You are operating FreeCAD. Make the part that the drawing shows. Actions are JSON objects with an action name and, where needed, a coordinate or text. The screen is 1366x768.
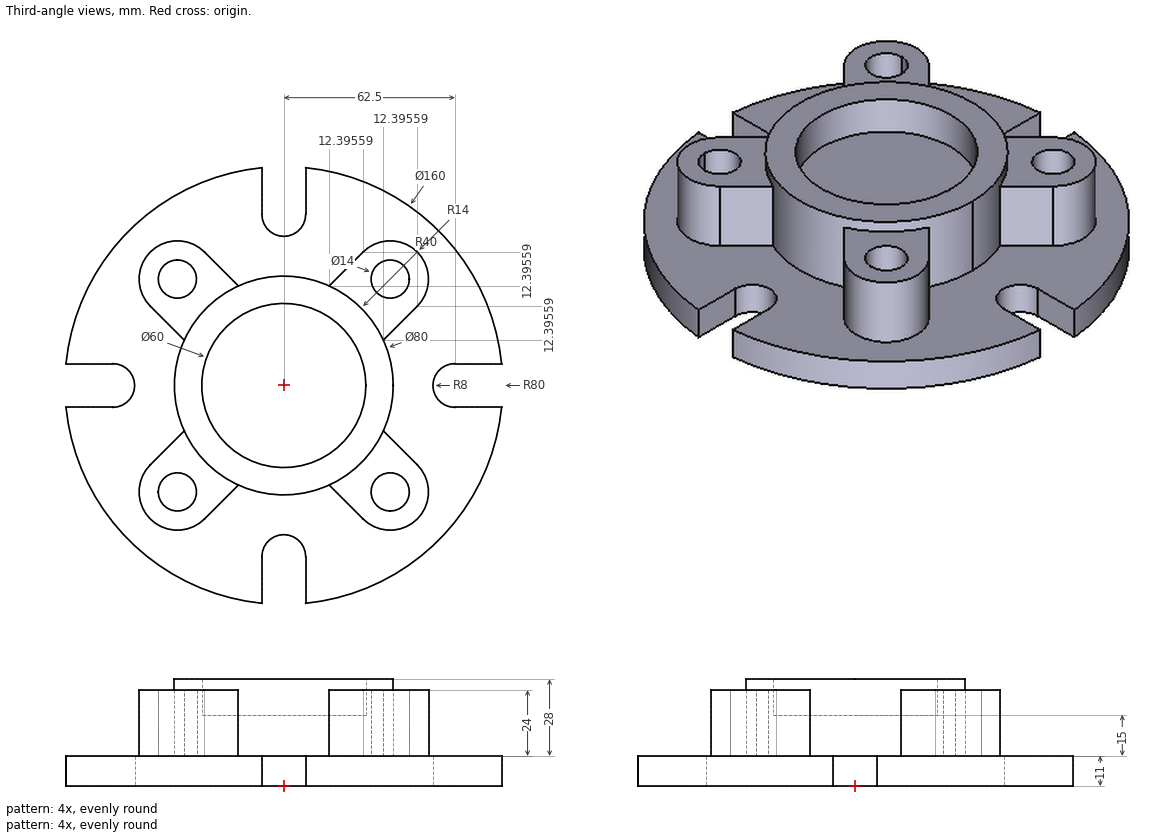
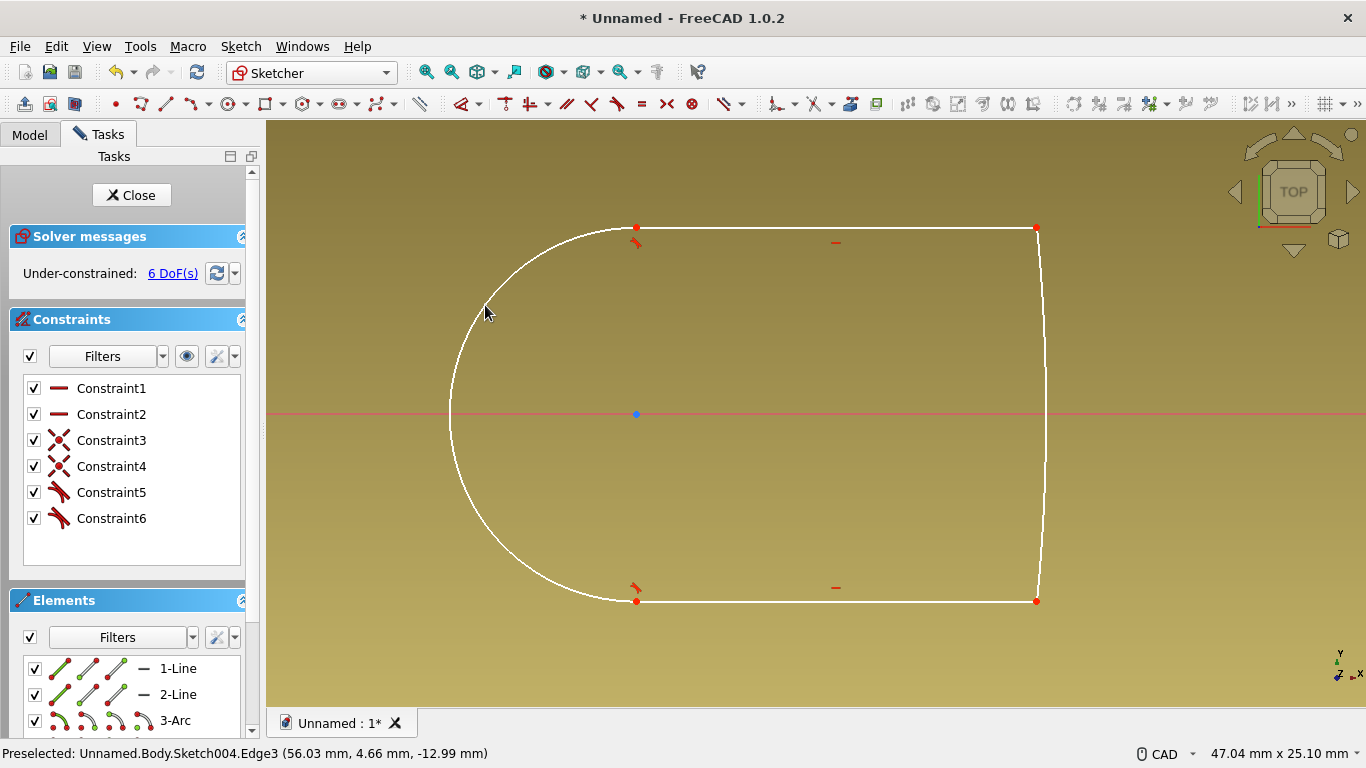
{"action": "scroll", "coordinate": [1125, 413], "scroll_direction": "down", "scroll_amount": 5}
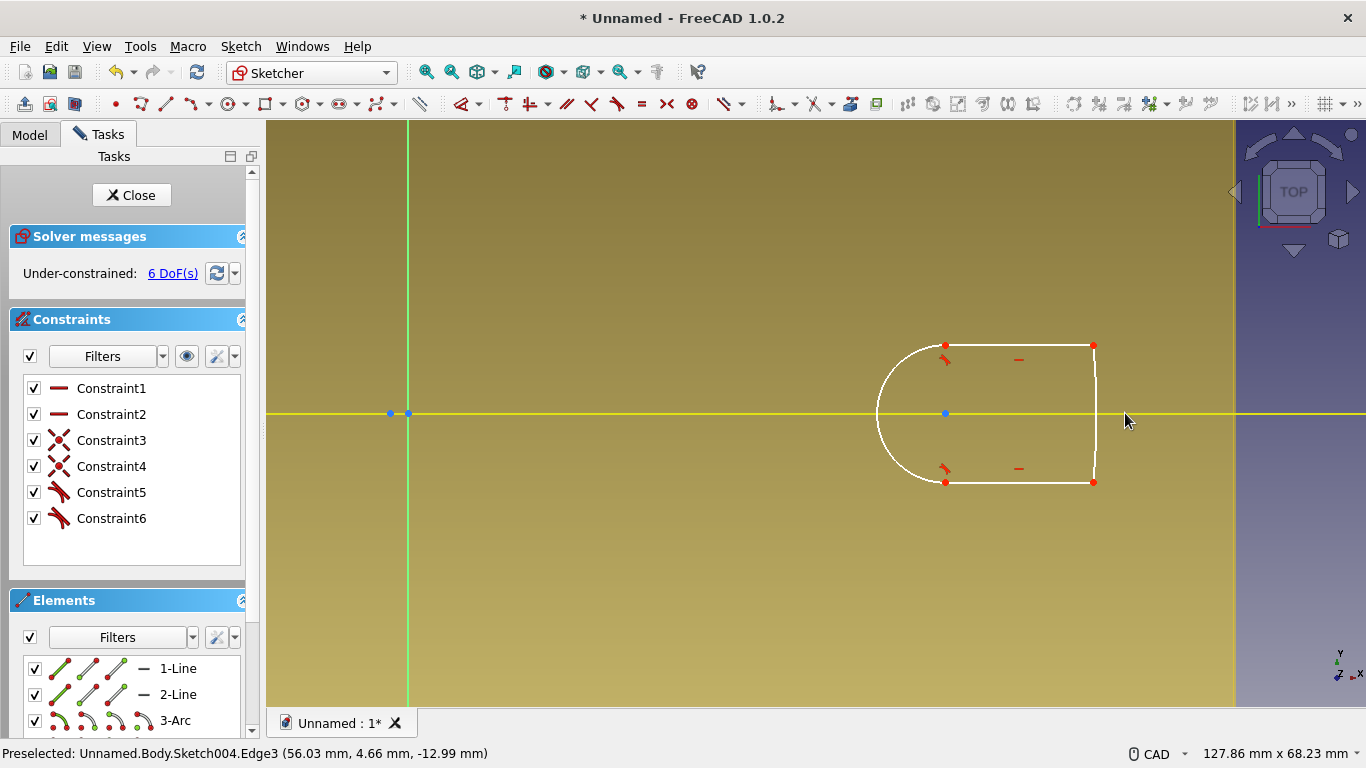
{"action": "left_click_drag", "start_coordinate": [380, 404], "coordinate": [418, 424]}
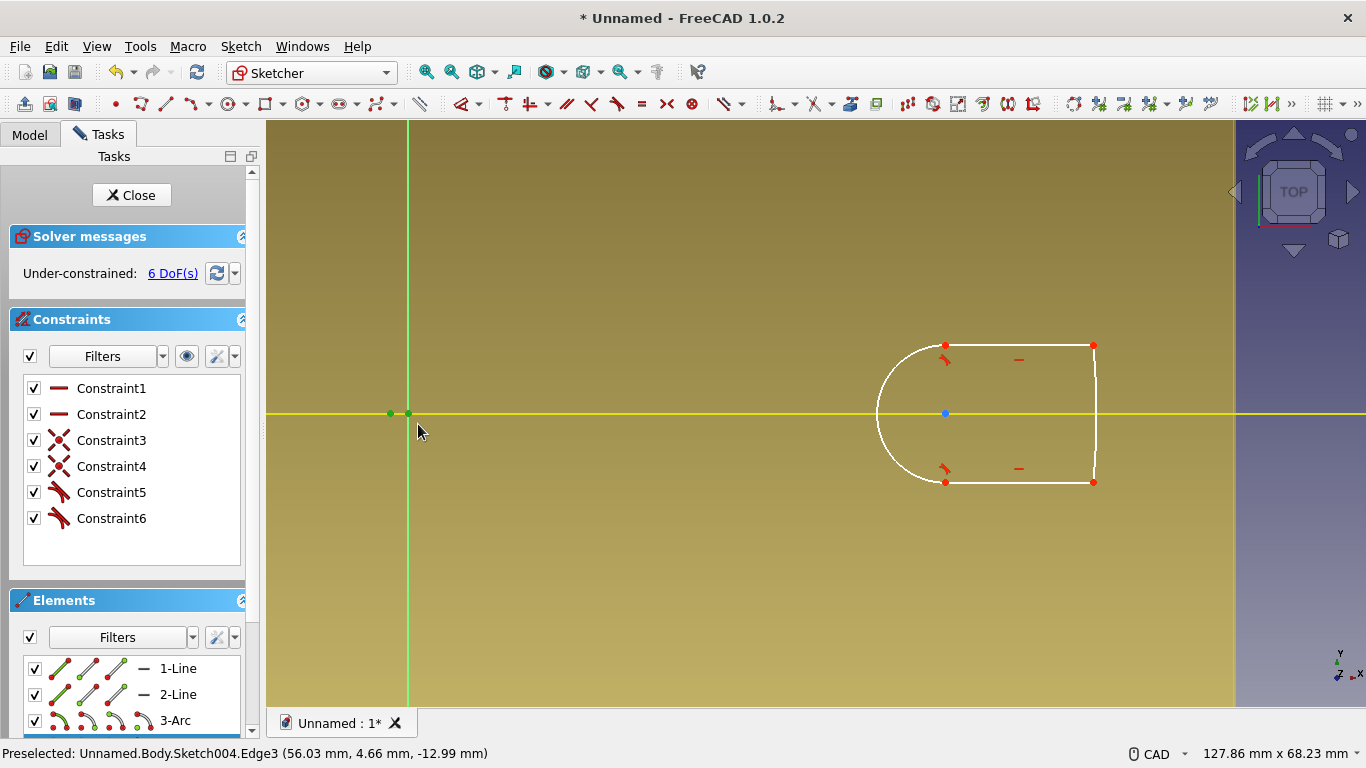
{"action": "key", "text": "c"}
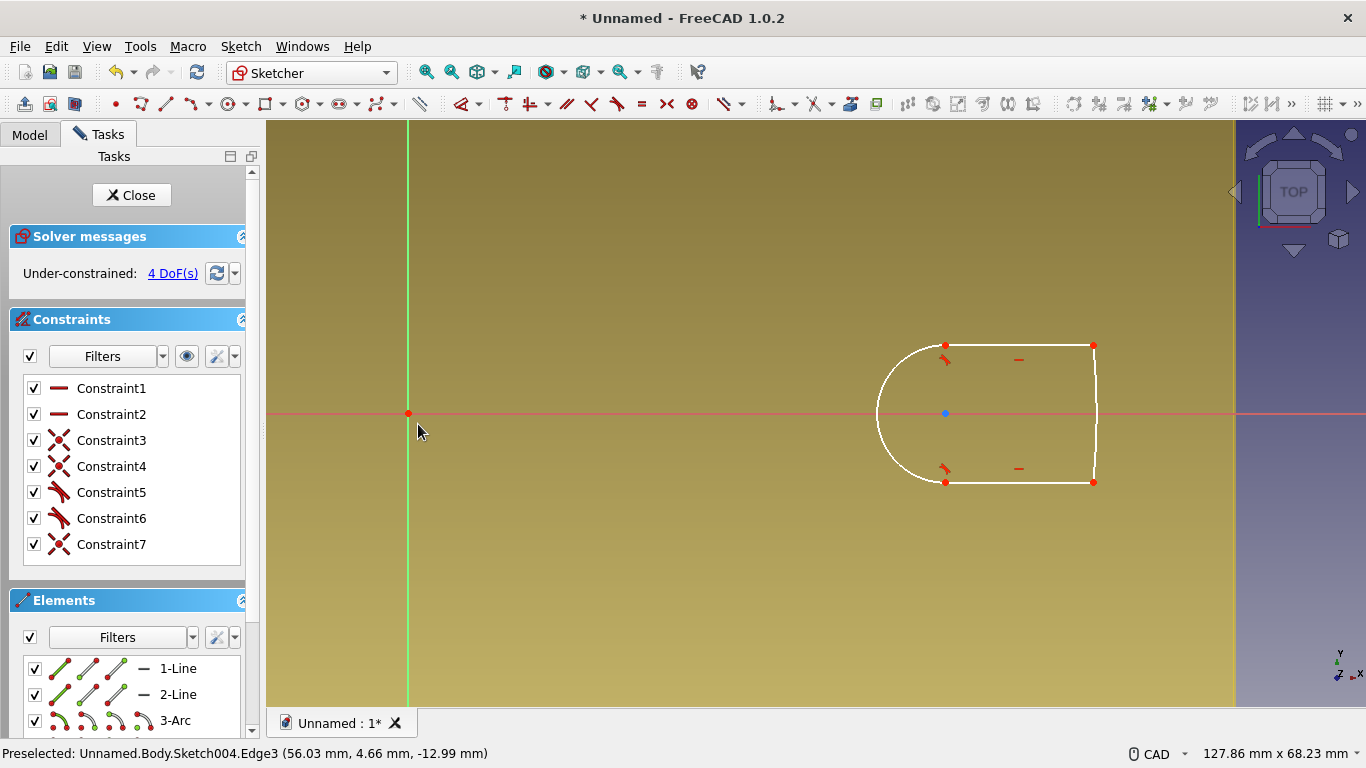
{"action": "left_click", "coordinate": [946, 414]}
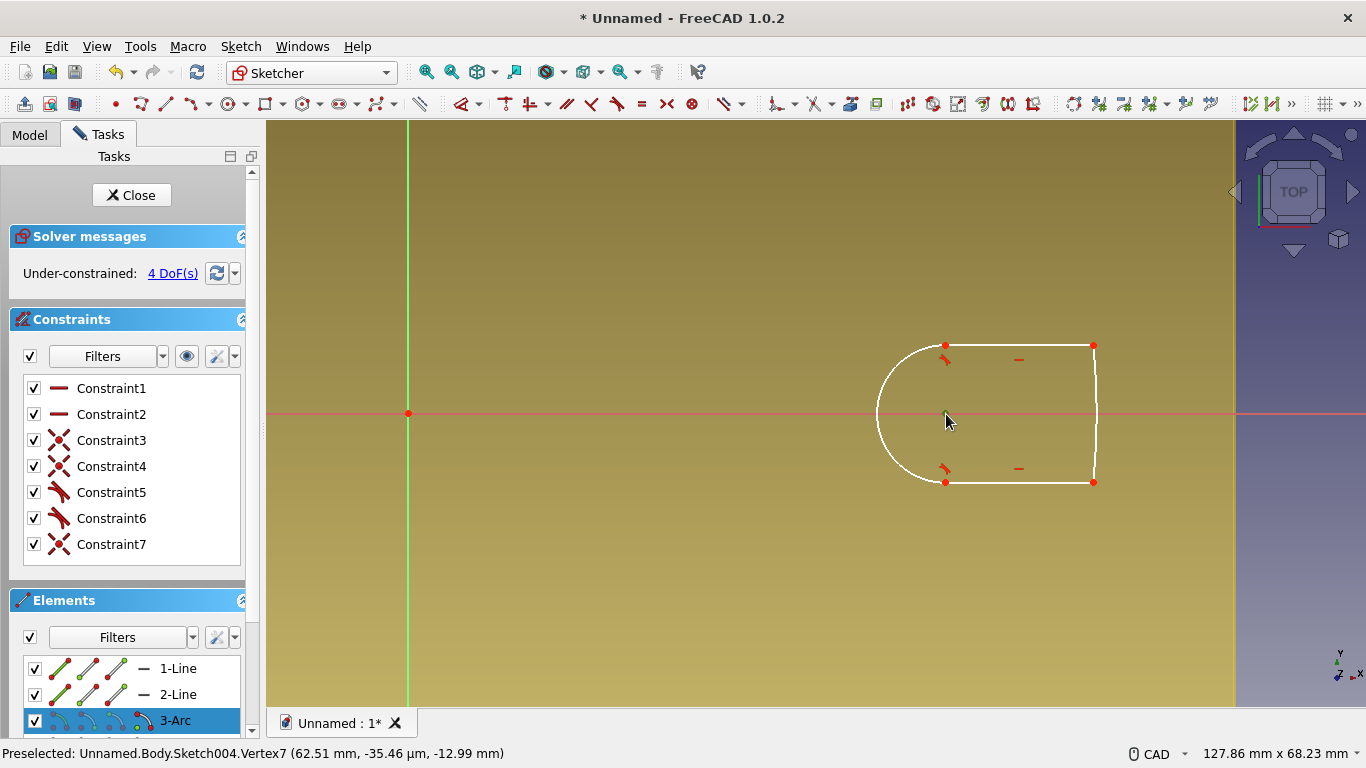
{"action": "left_click", "coordinate": [359, 414]}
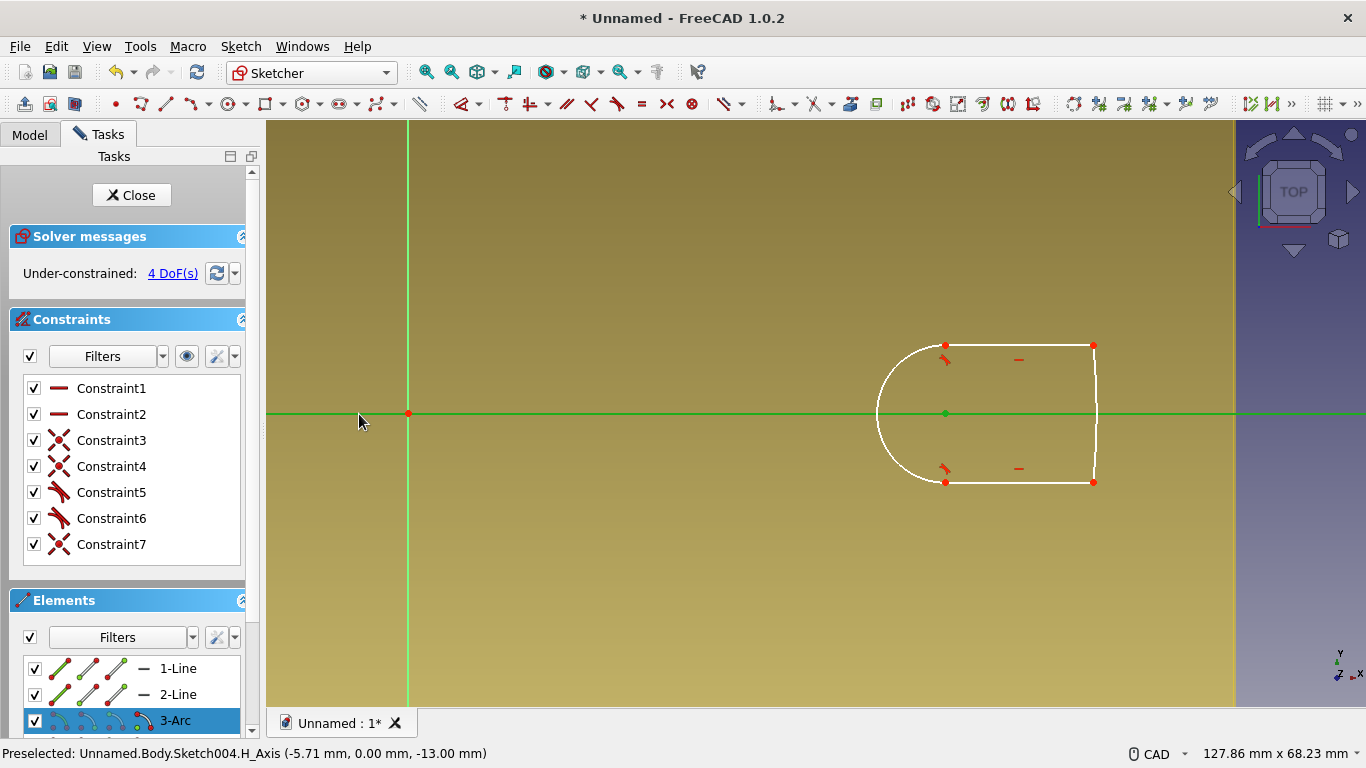
{"action": "key", "text": "c"}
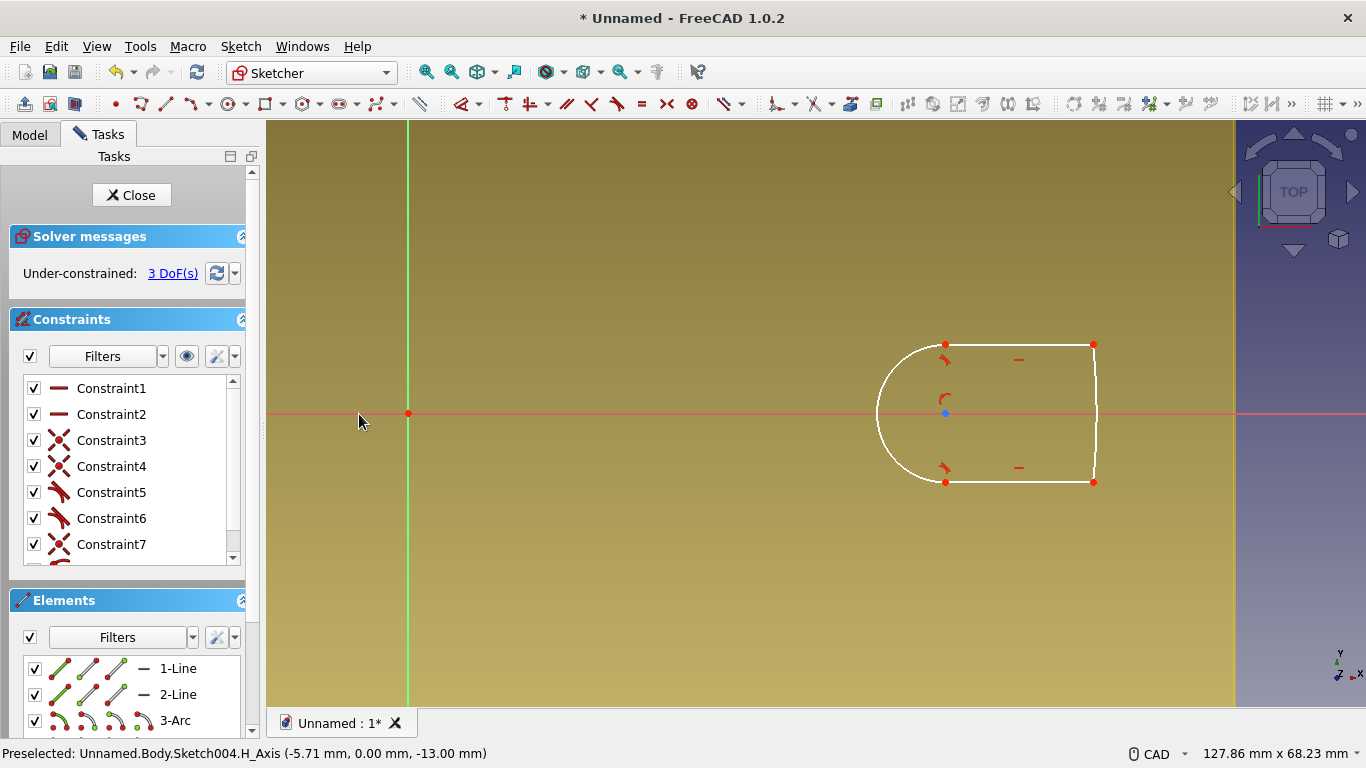
{"action": "left_click", "coordinate": [460, 104]}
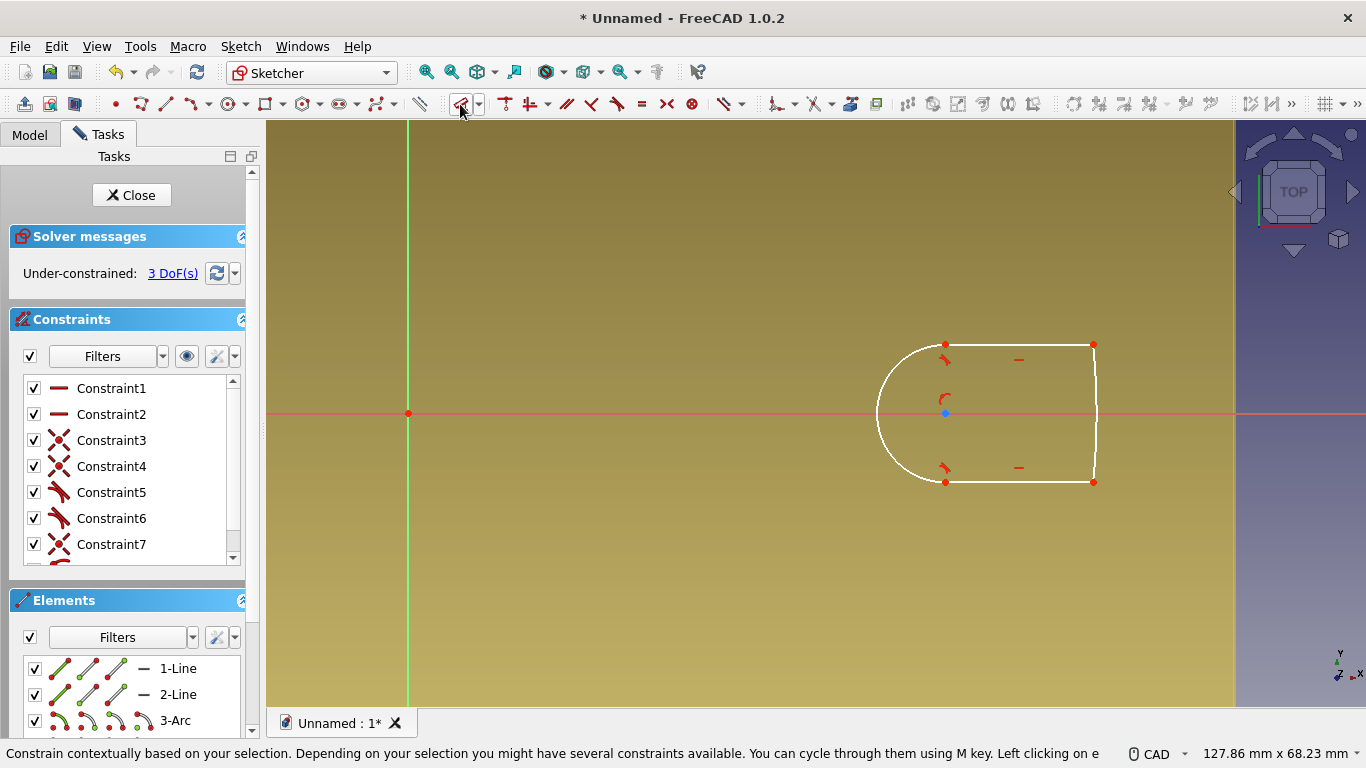
{"action": "left_click", "coordinate": [890, 373]}
{"action": "left_click", "coordinate": [864, 354]}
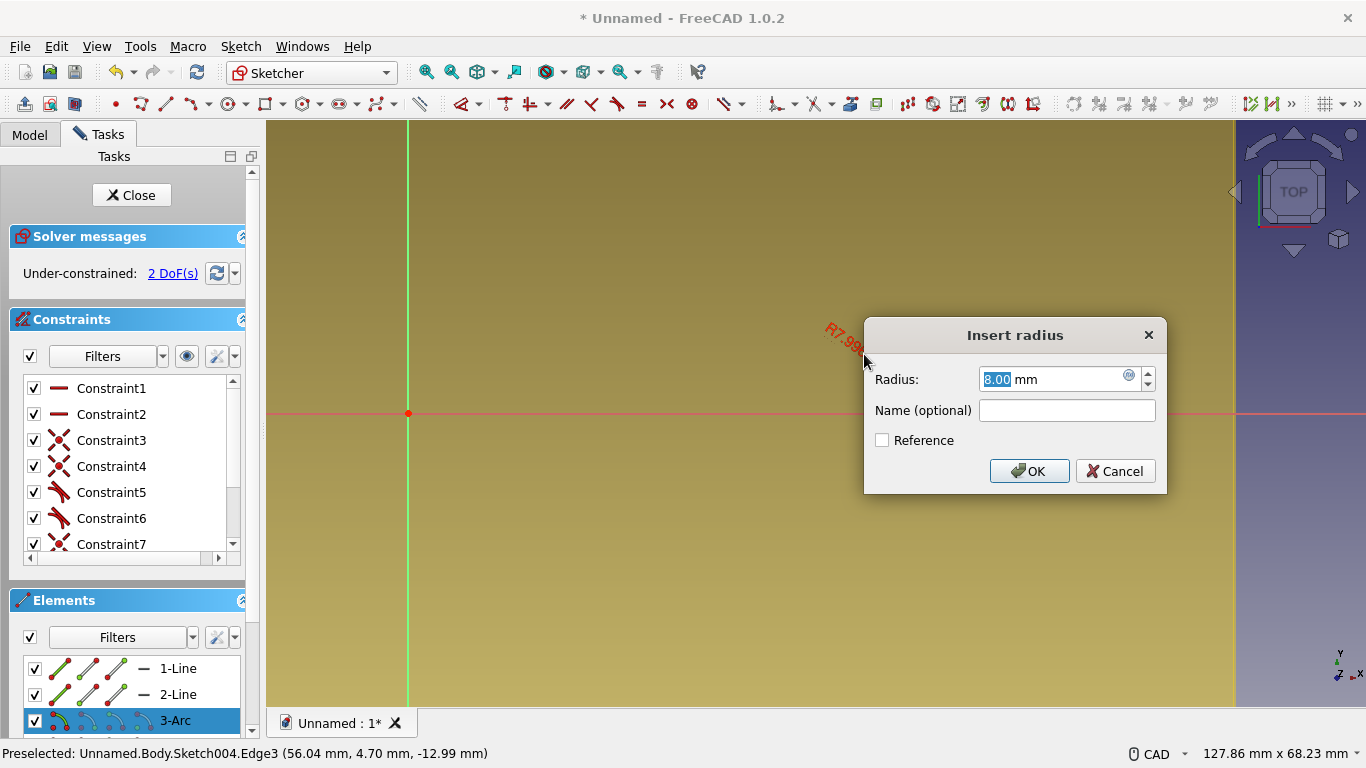
{"action": "type", "text": "8"}
{"action": "key", "text": "Return"}